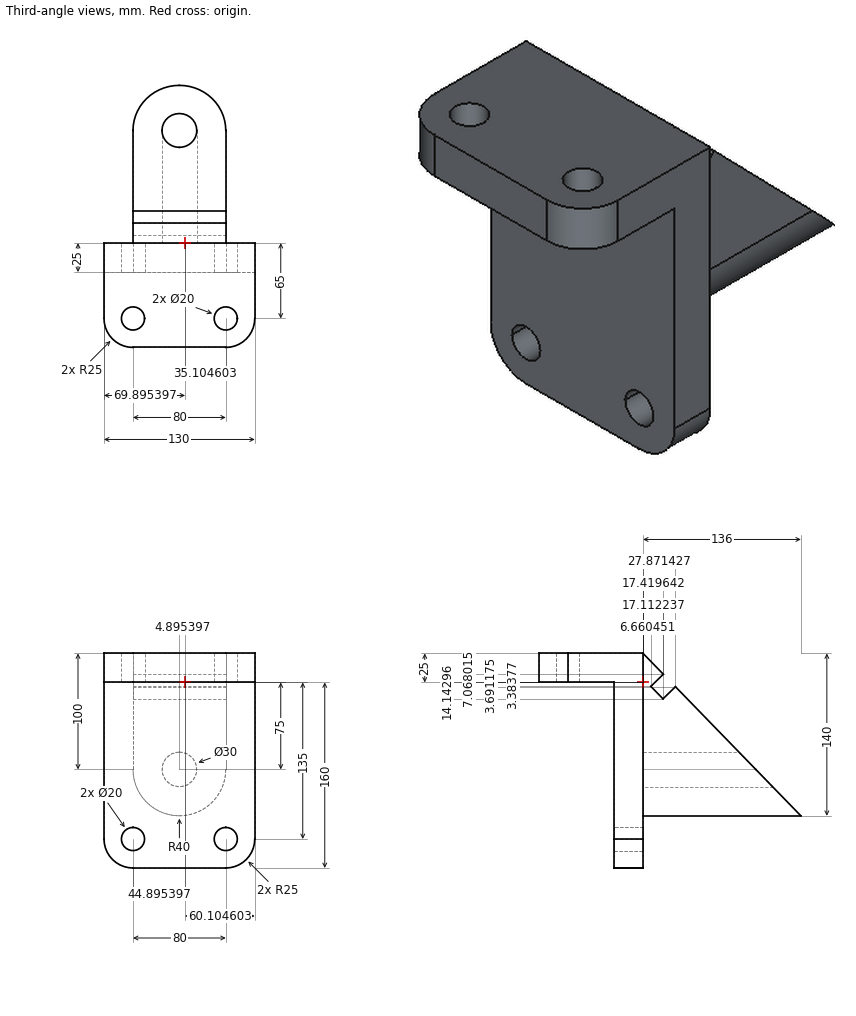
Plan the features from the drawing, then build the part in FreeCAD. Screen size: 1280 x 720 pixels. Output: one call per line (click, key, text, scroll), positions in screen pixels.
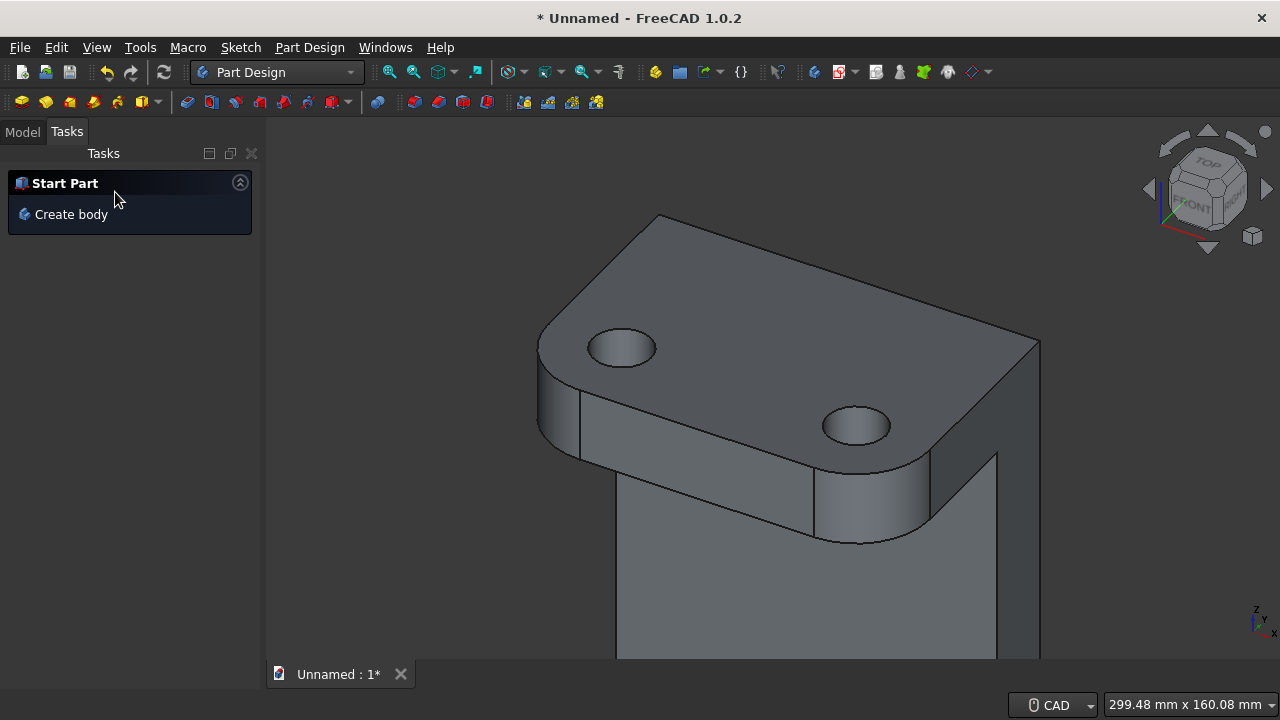
click(390, 72)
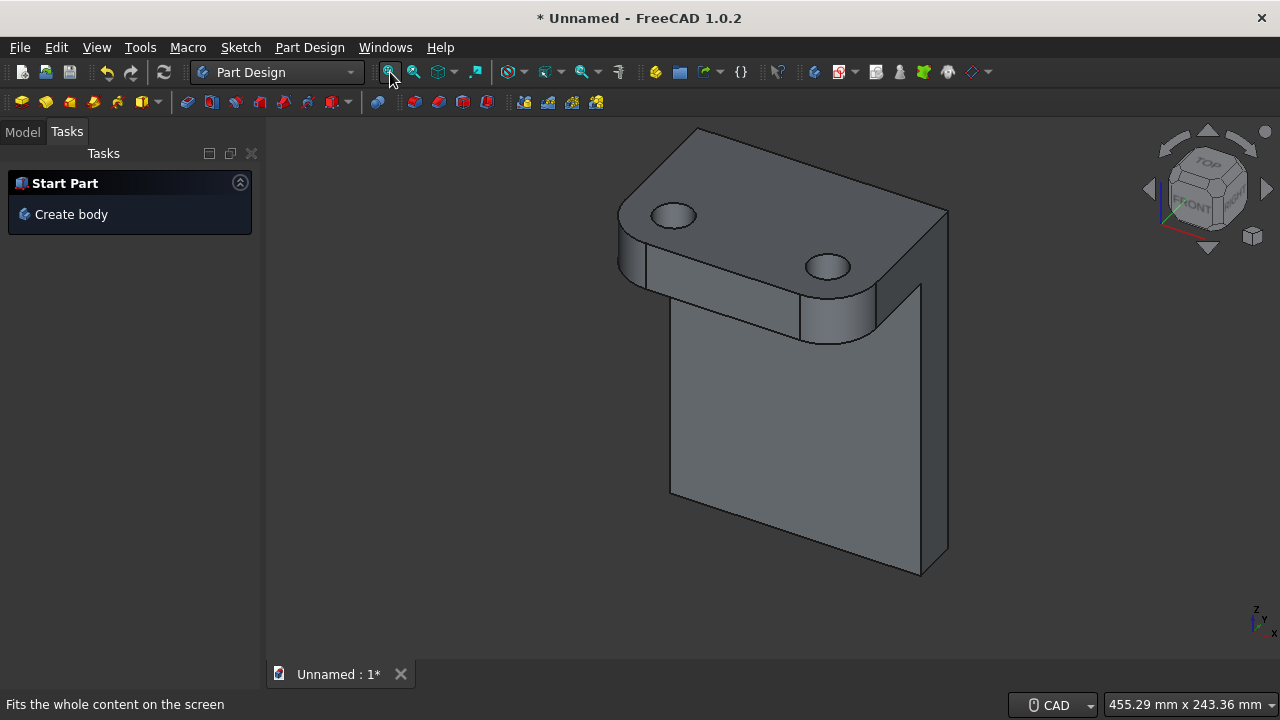
key(4)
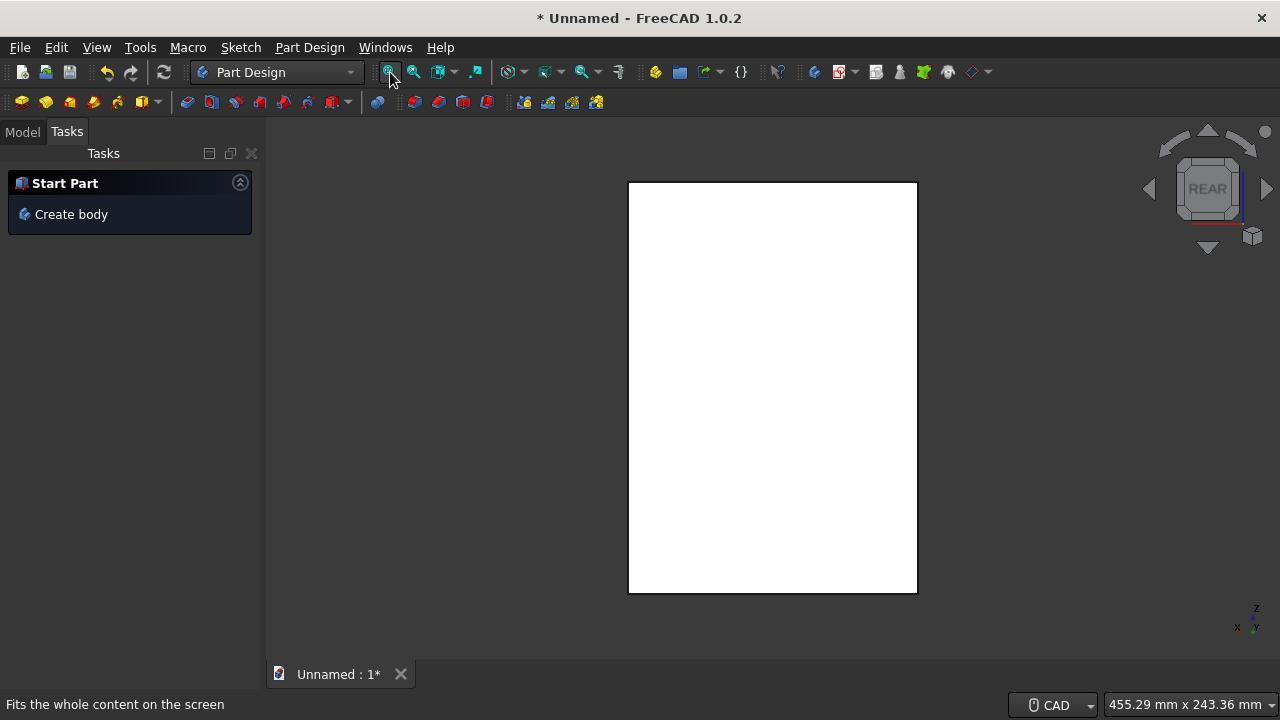
click(773, 328)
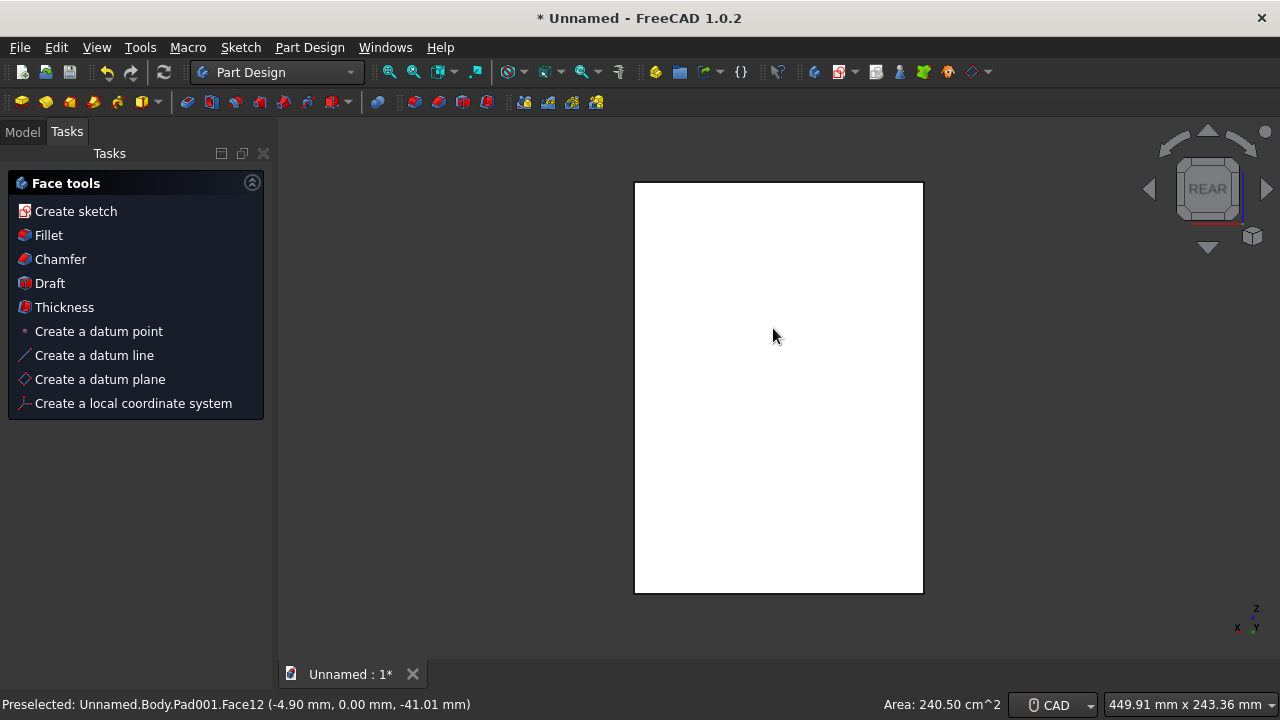
click(840, 72)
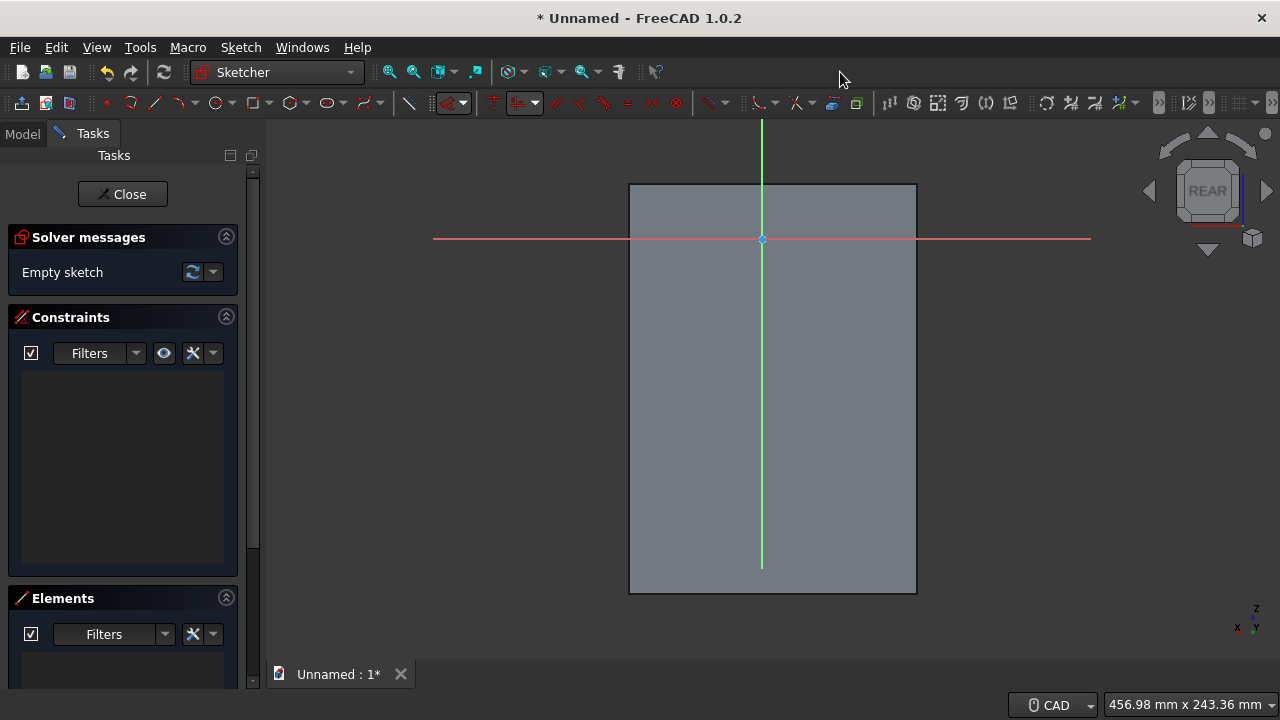
click(132, 104)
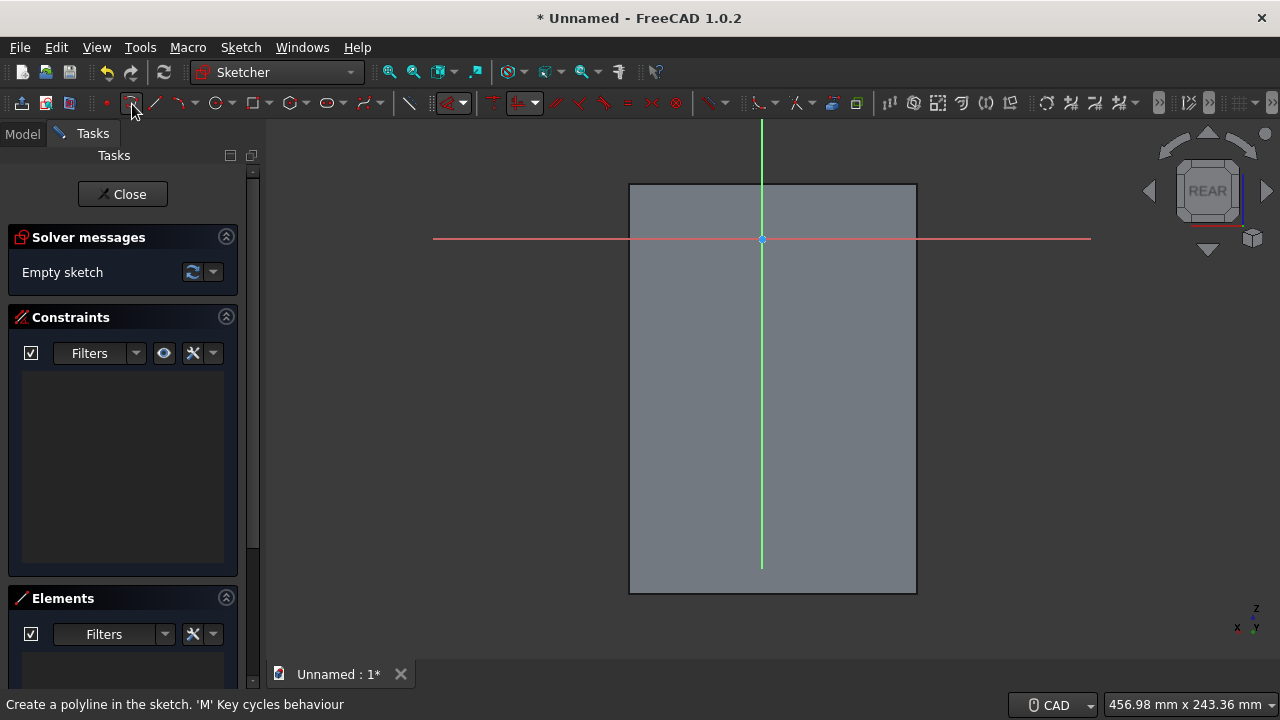
click(629, 539)
click(629, 594)
click(684, 594)
right_click(684, 594)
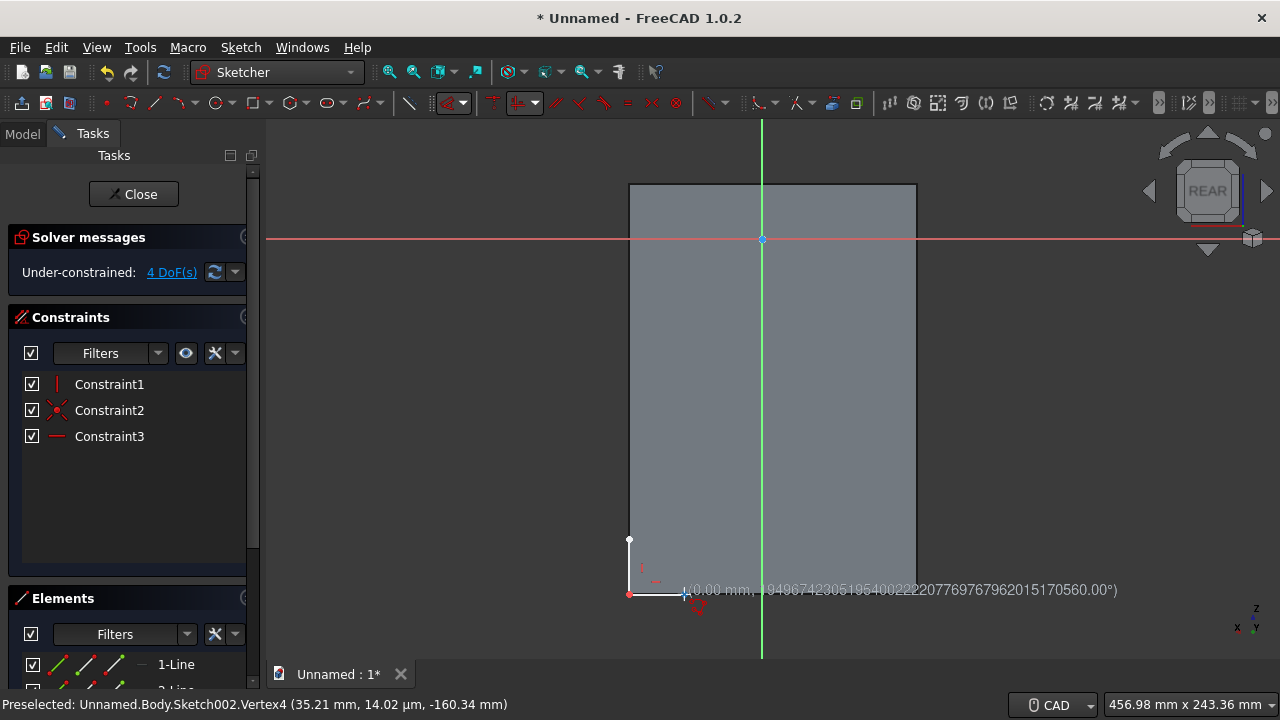
click(180, 104)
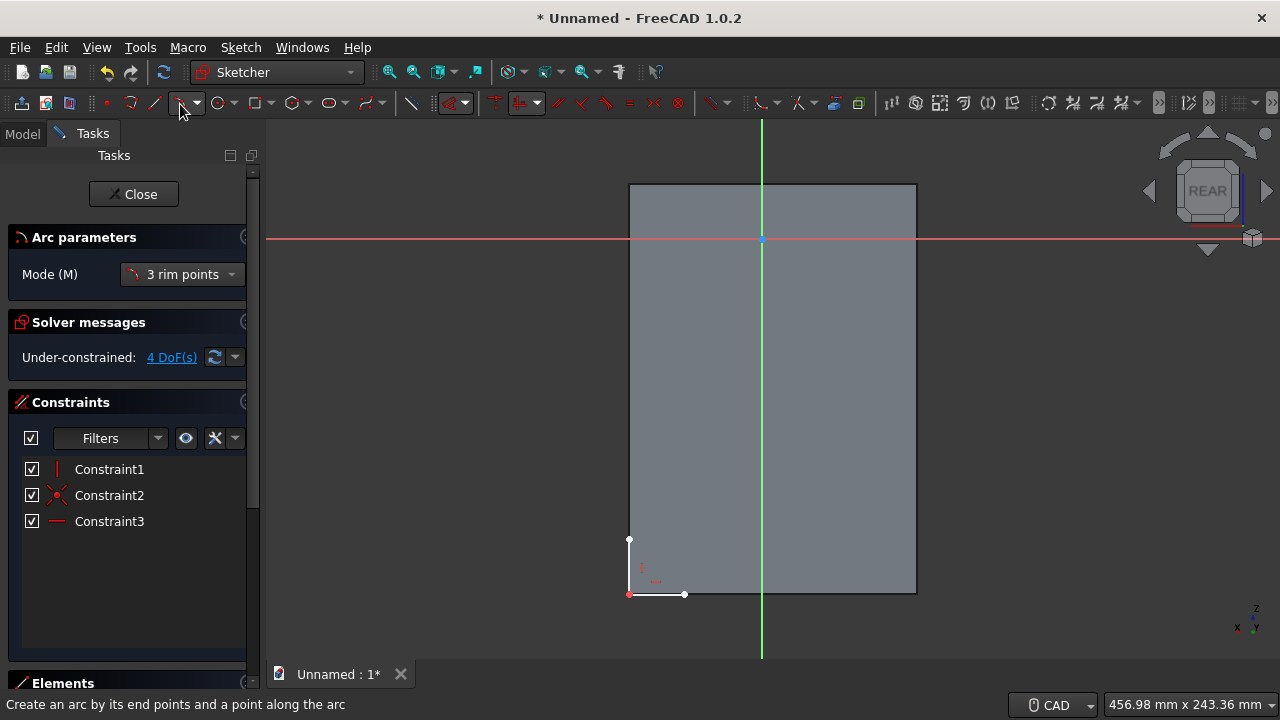
click(684, 595)
click(629, 540)
click(645, 578)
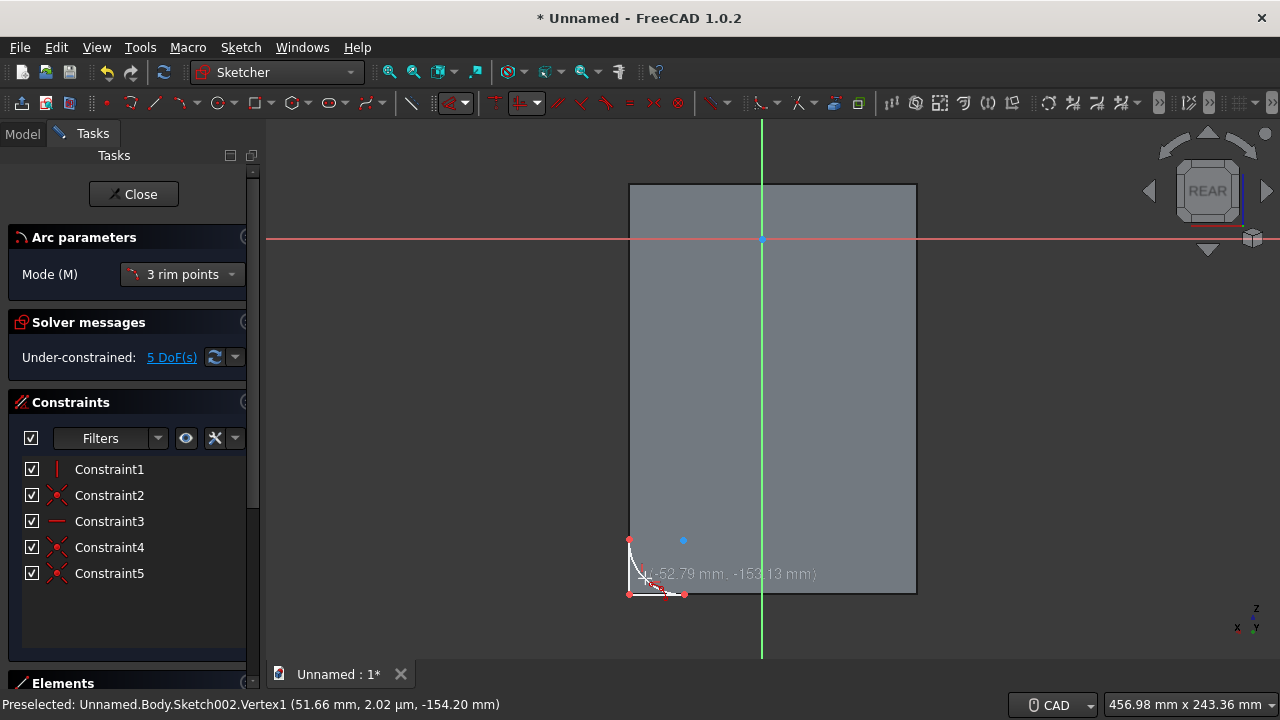
click(132, 104)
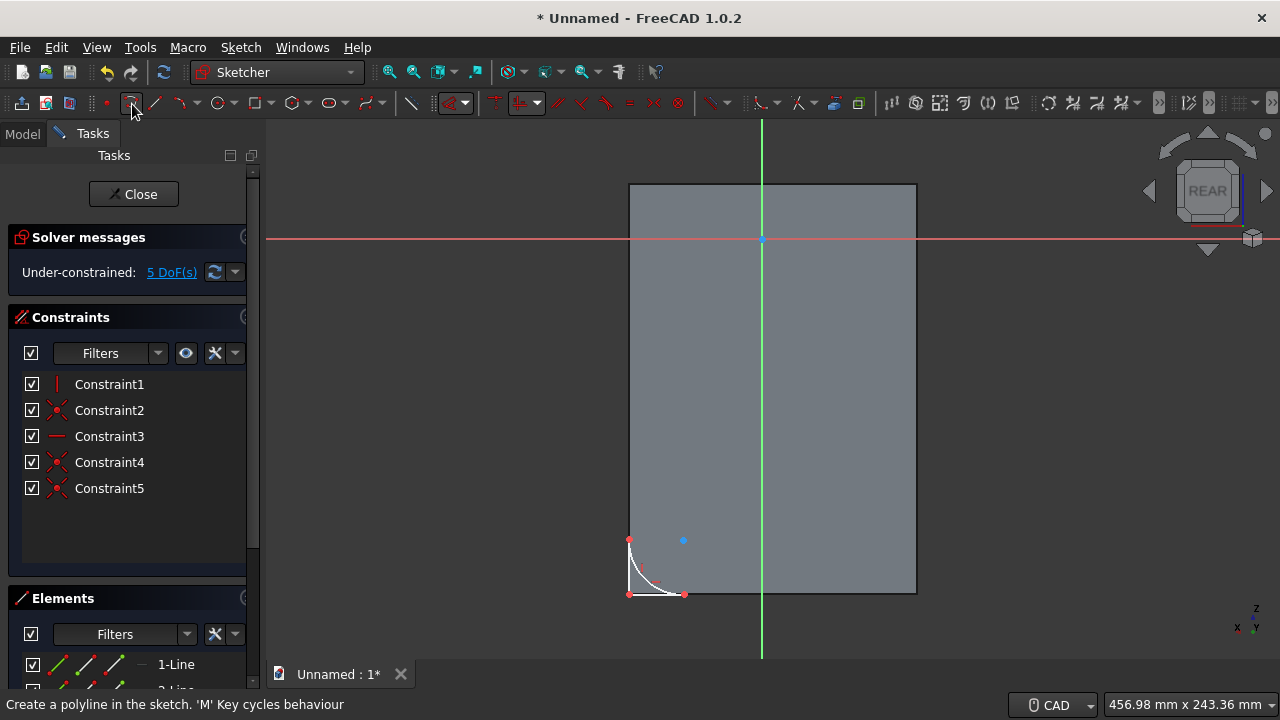
click(862, 594)
click(917, 594)
click(917, 539)
right_click(917, 539)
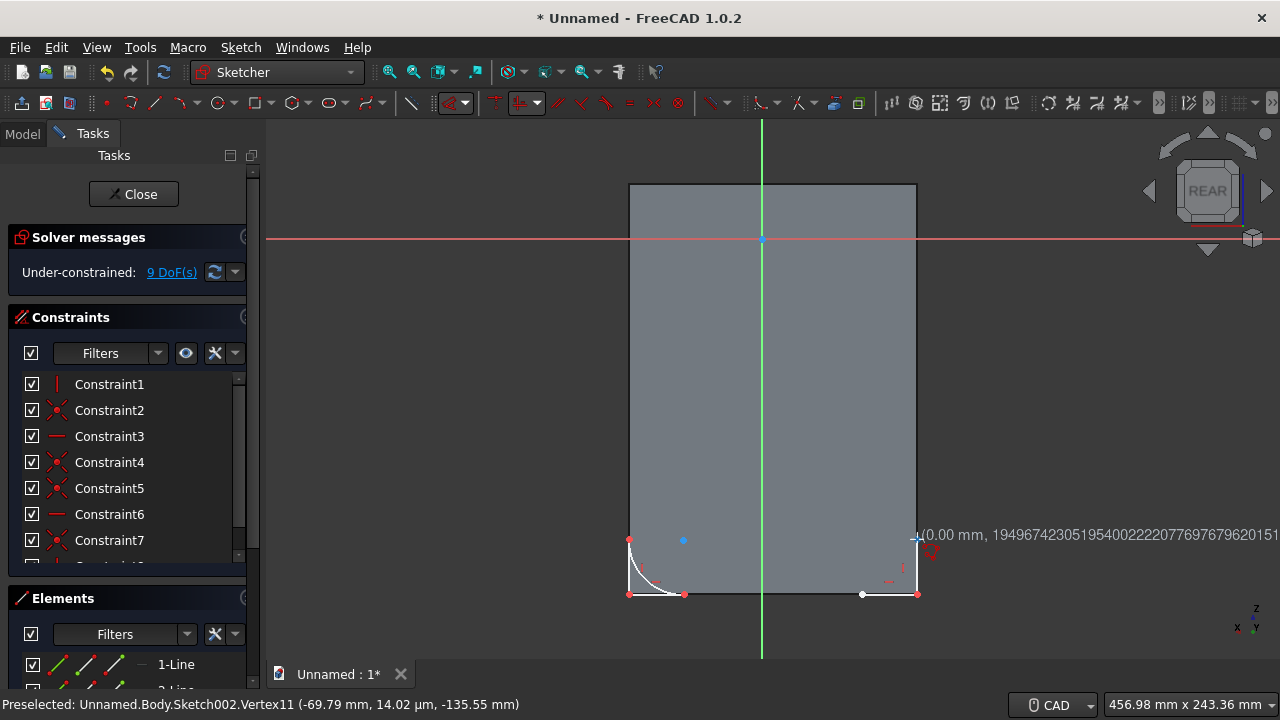
key(g)
key(3)
key(a)